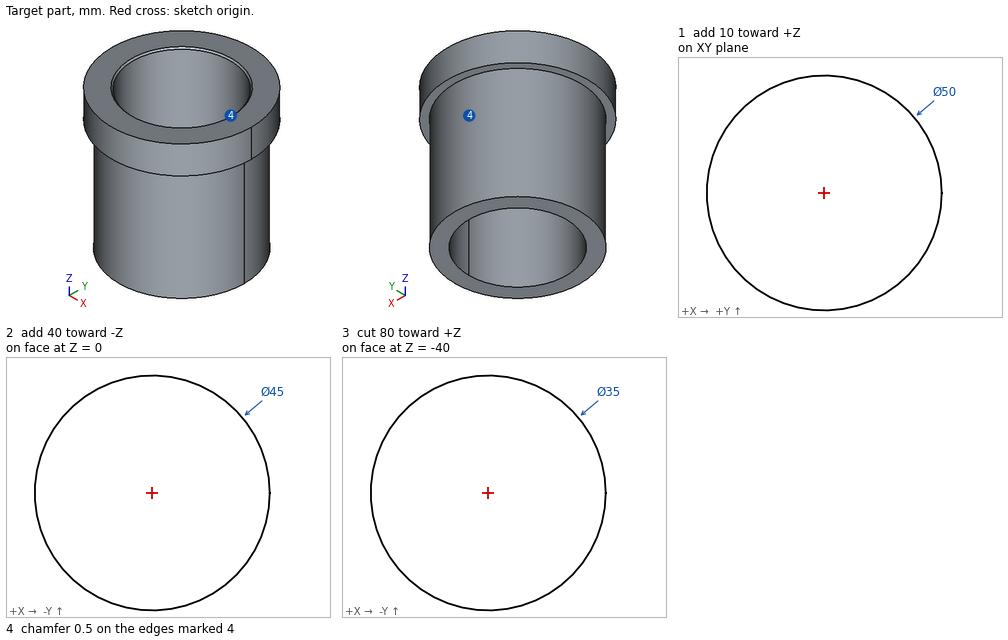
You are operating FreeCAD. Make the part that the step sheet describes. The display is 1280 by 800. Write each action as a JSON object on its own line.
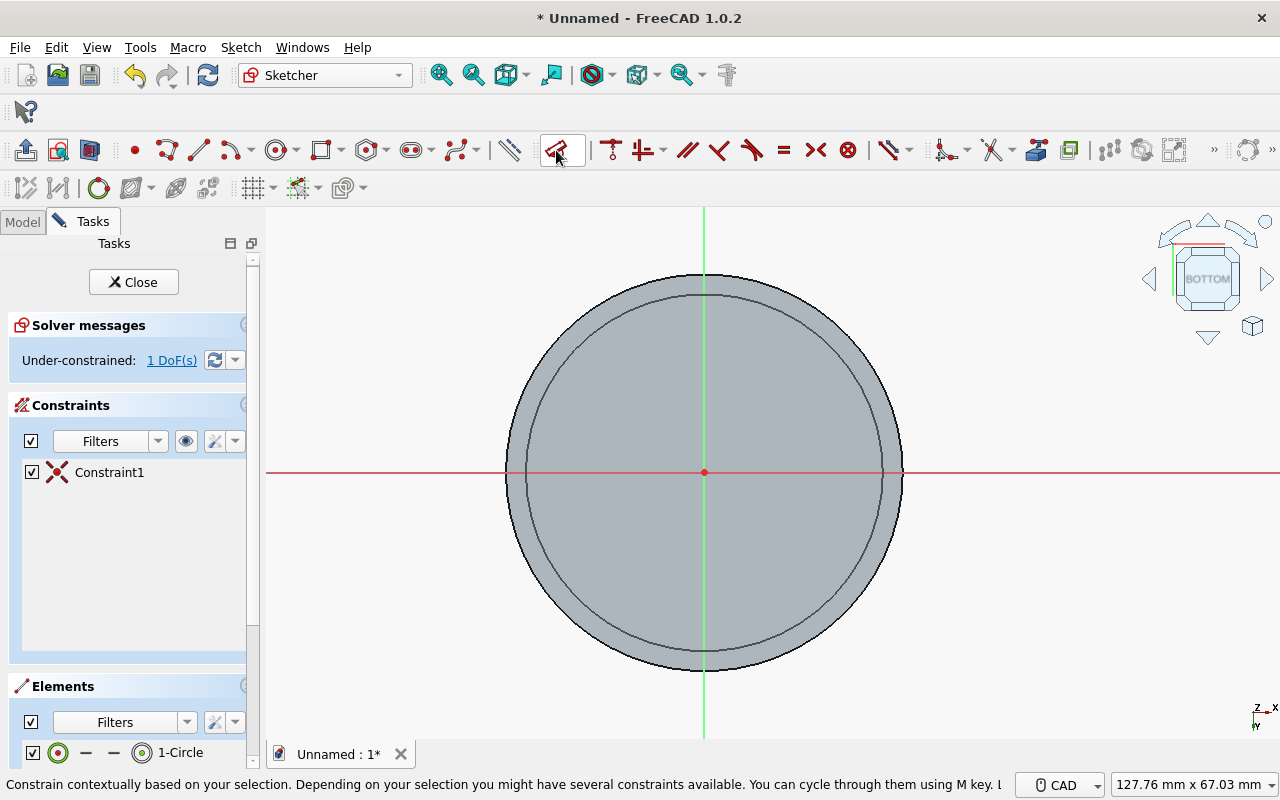
{"action": "left_click", "coordinate": [830, 346]}
{"action": "left_click", "coordinate": [853, 323]}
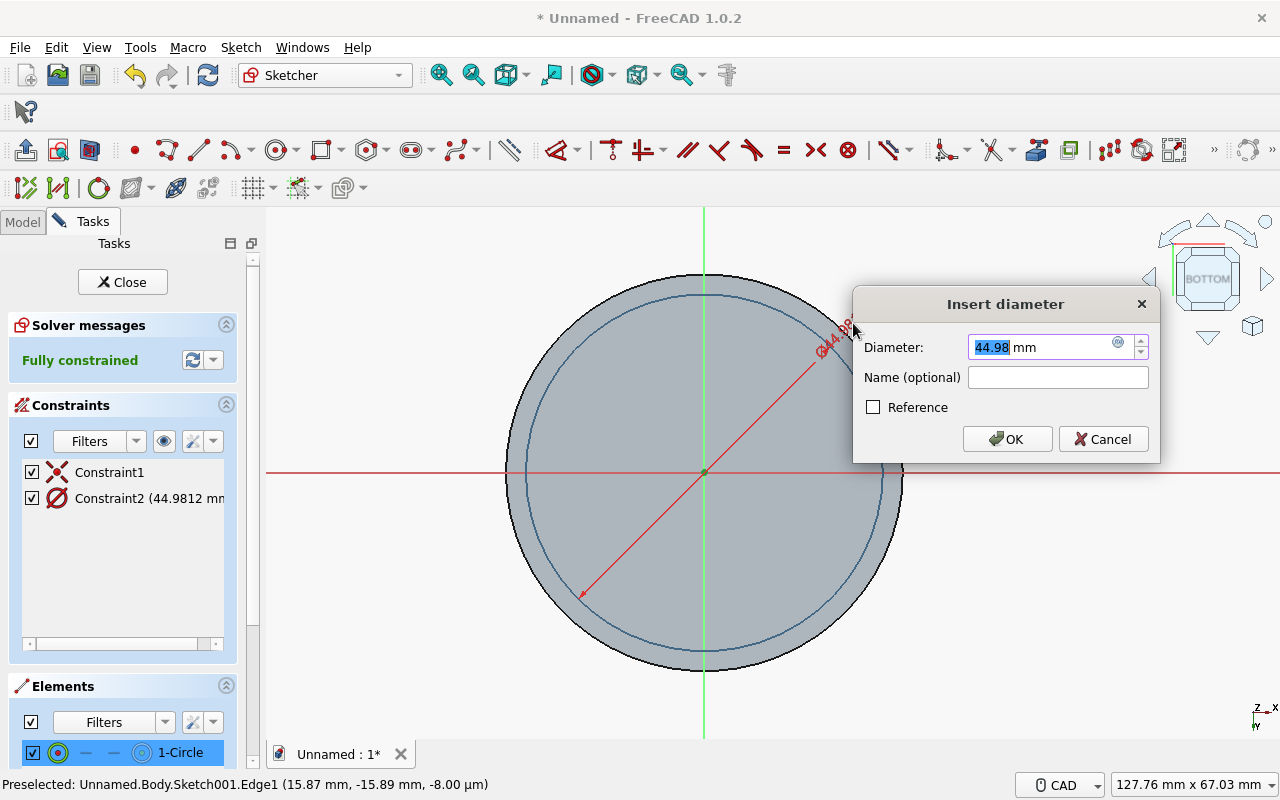
{"action": "type", "text": "45"}
{"action": "key", "text": "Return"}
{"action": "key", "text": "Escape"}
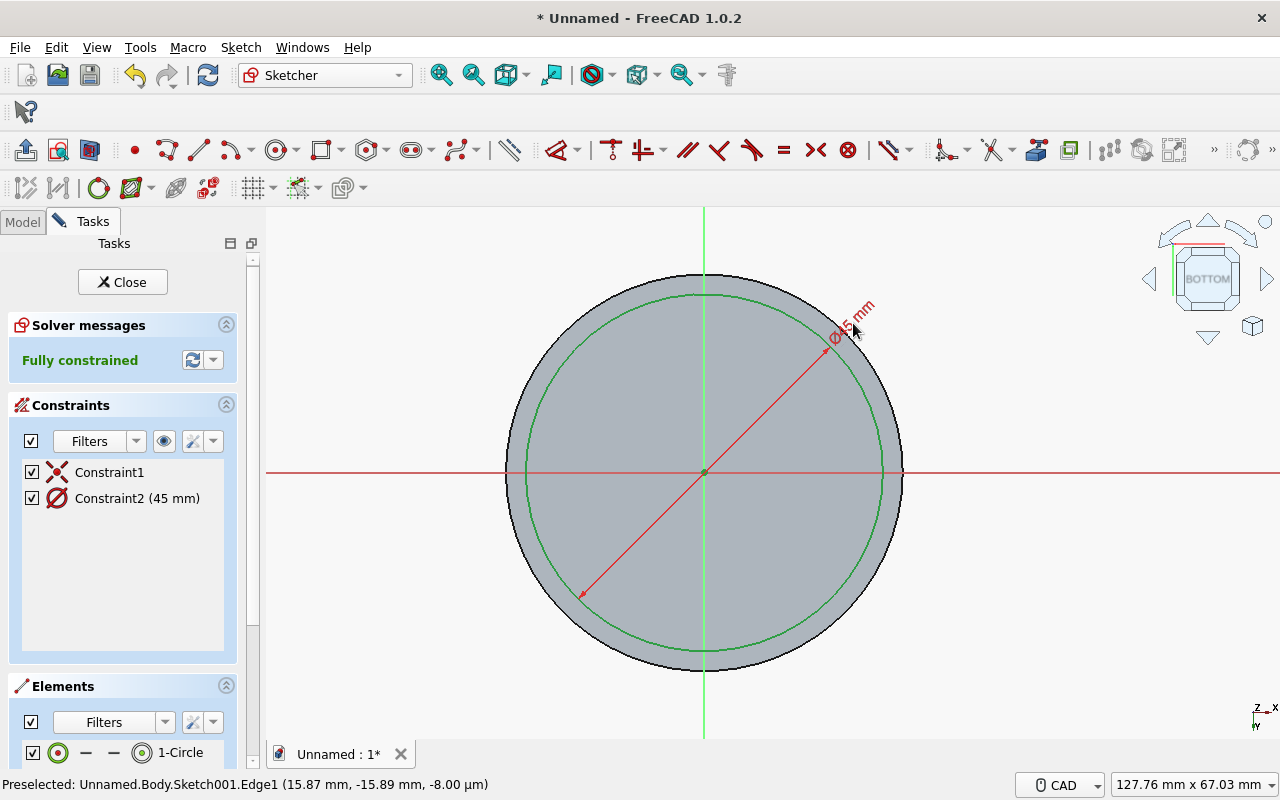
{"action": "left_click", "coordinate": [123, 282]}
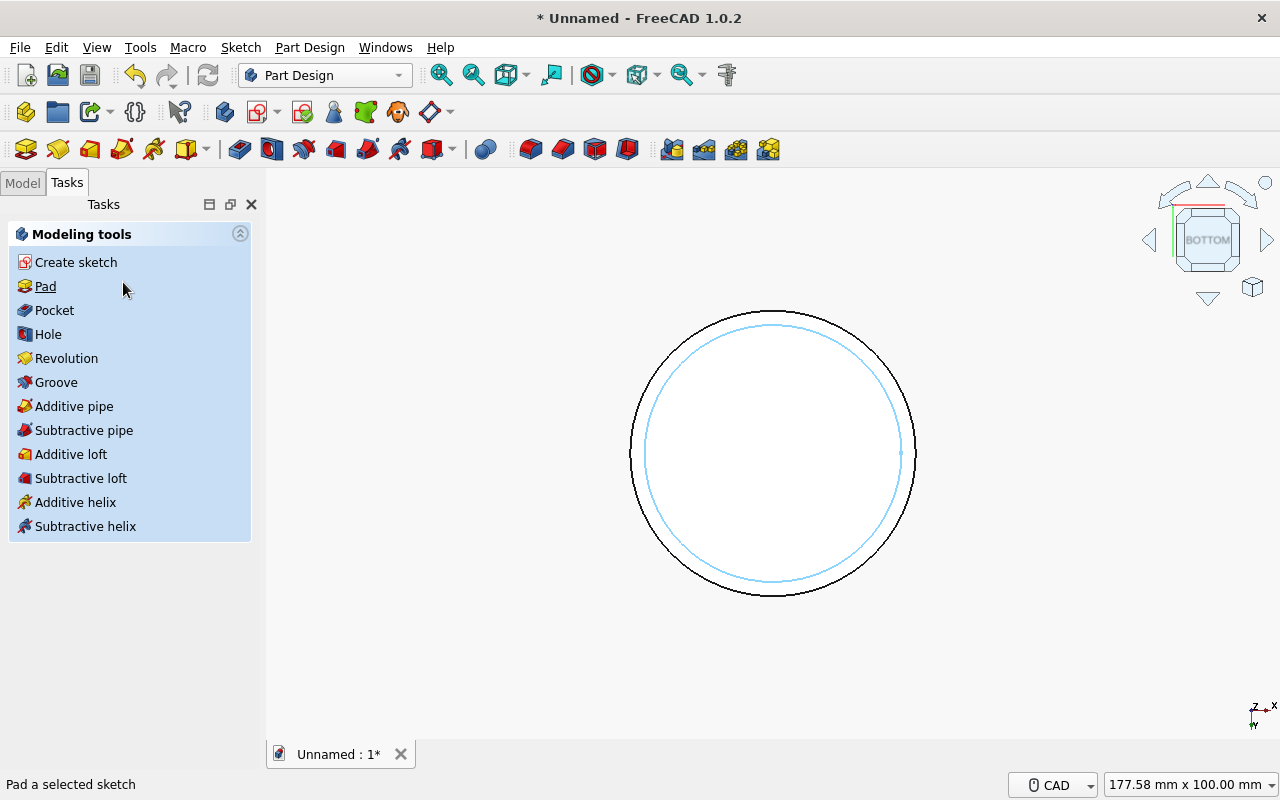
{"action": "left_click", "coordinate": [26, 150]}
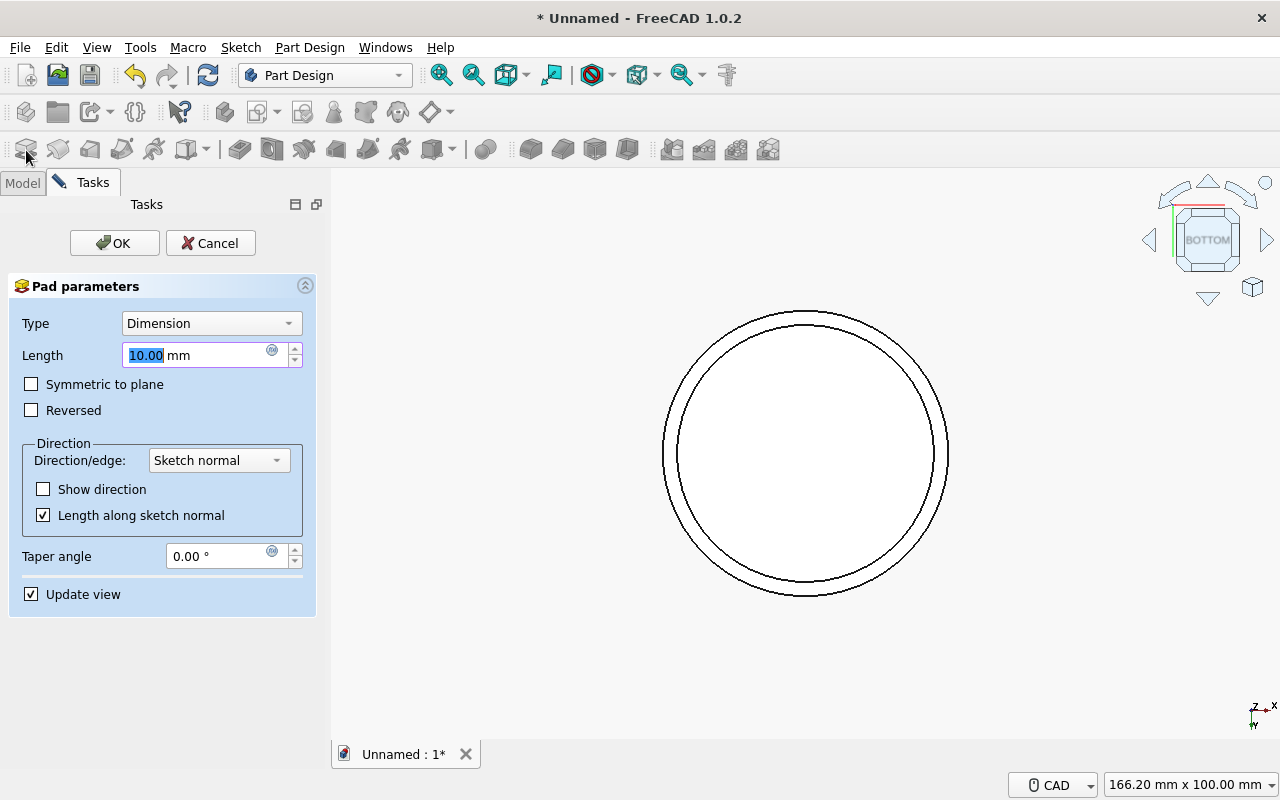
{"action": "type", "text": "40"}
{"action": "key", "text": "Tab"}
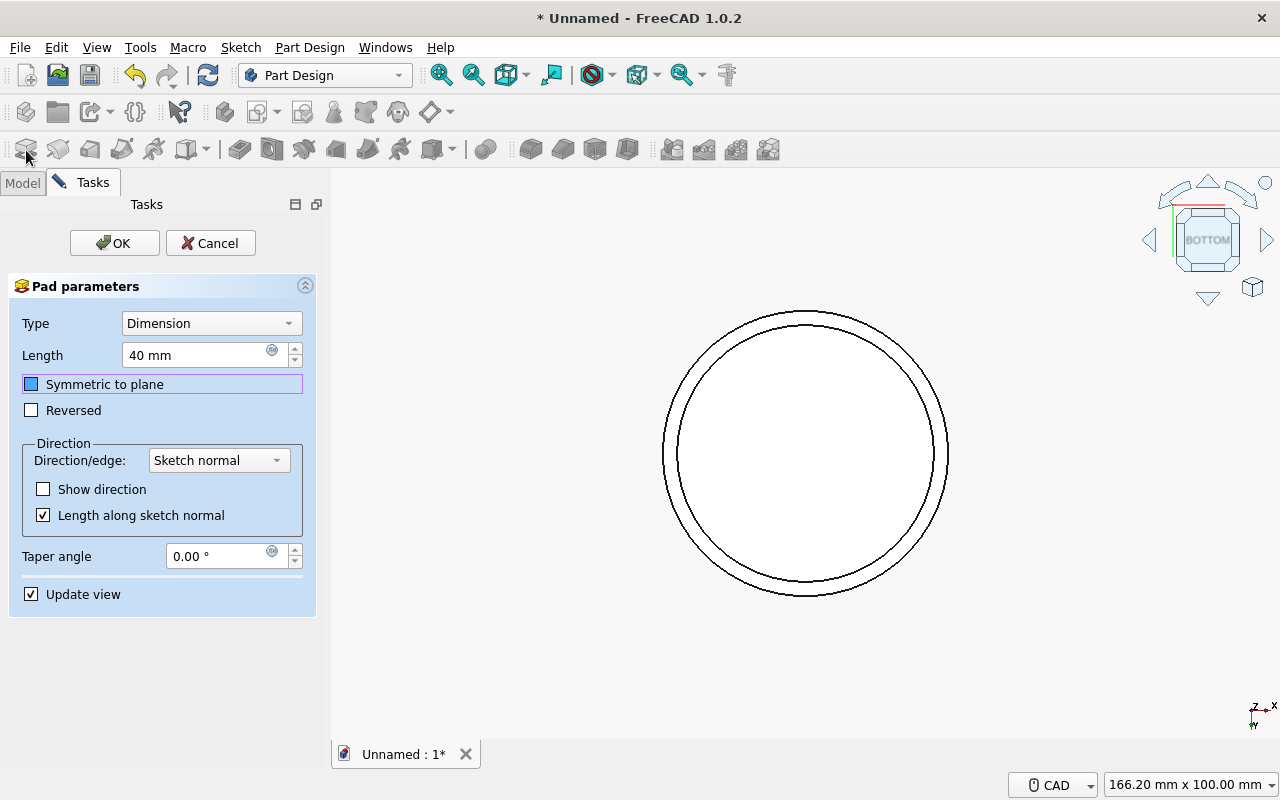
{"action": "left_click", "coordinate": [115, 243]}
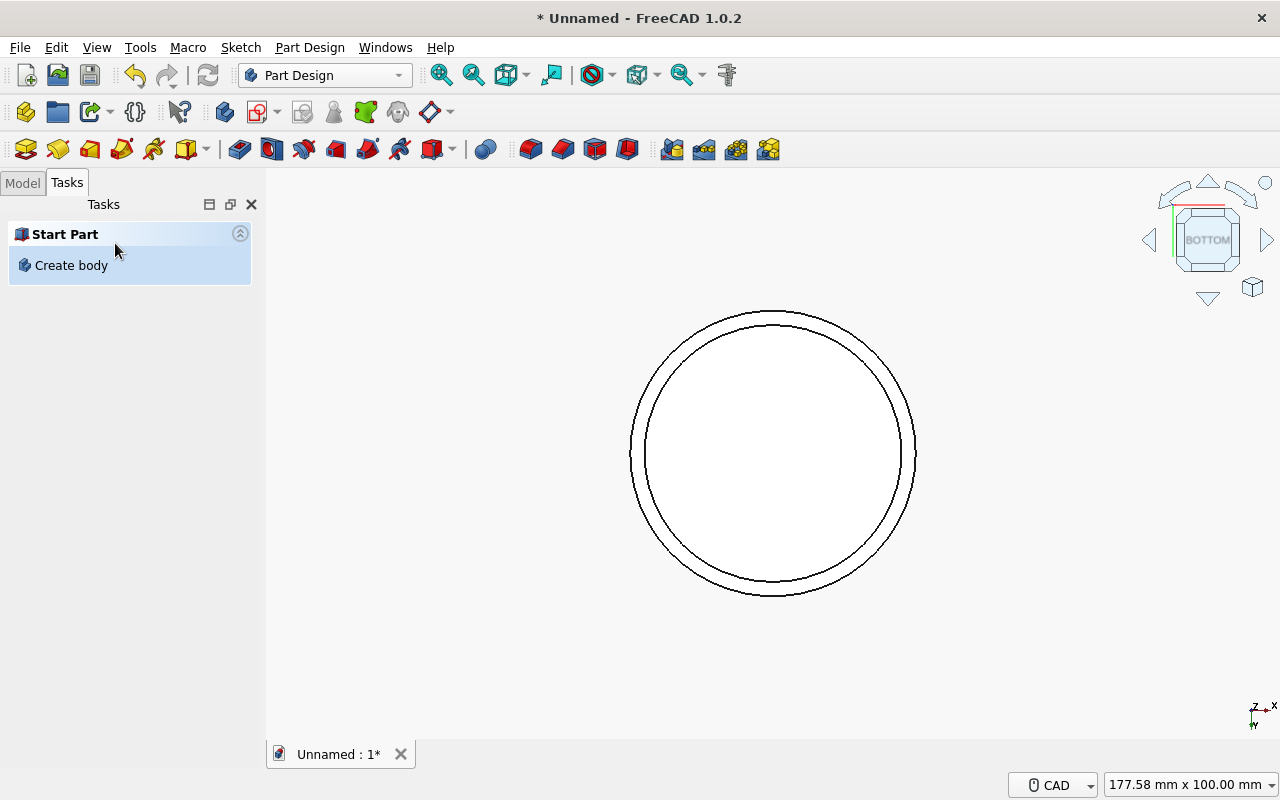
{"action": "left_click", "coordinate": [773, 453]}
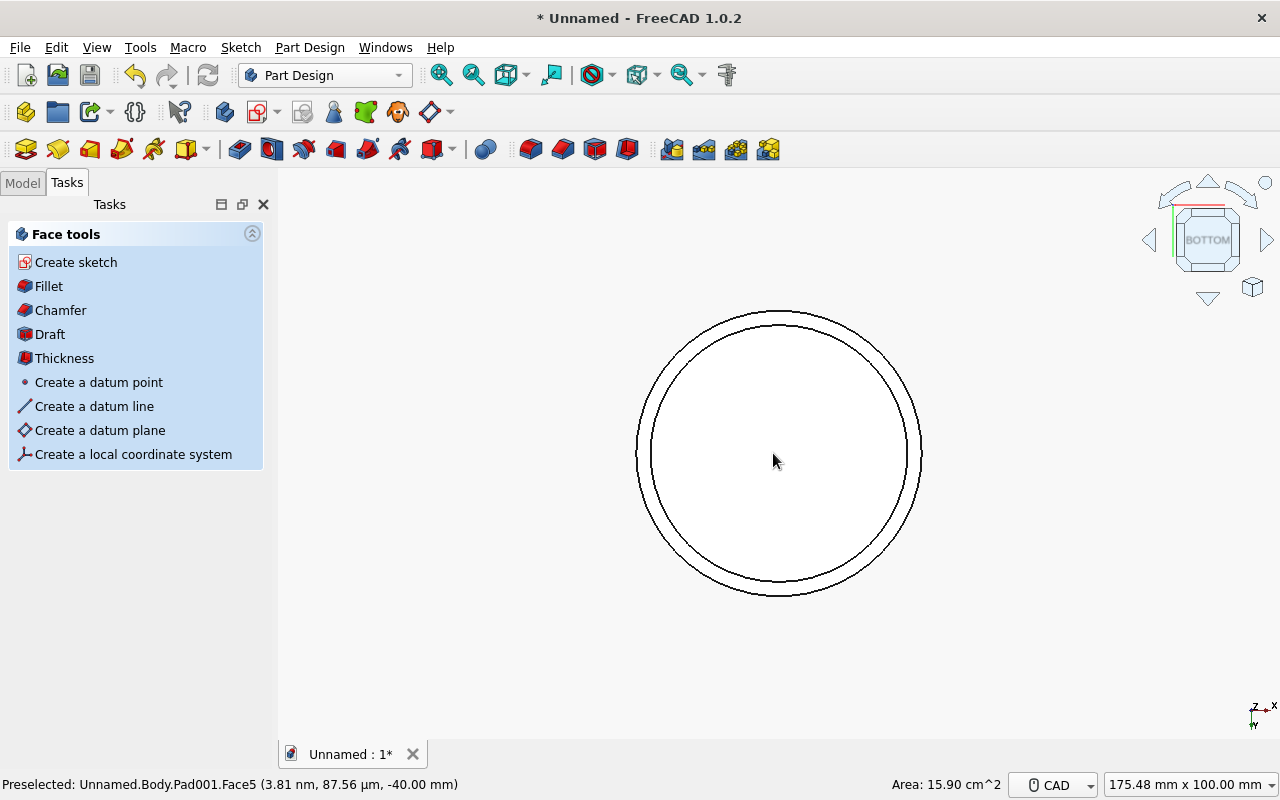
{"action": "left_click", "coordinate": [258, 112]}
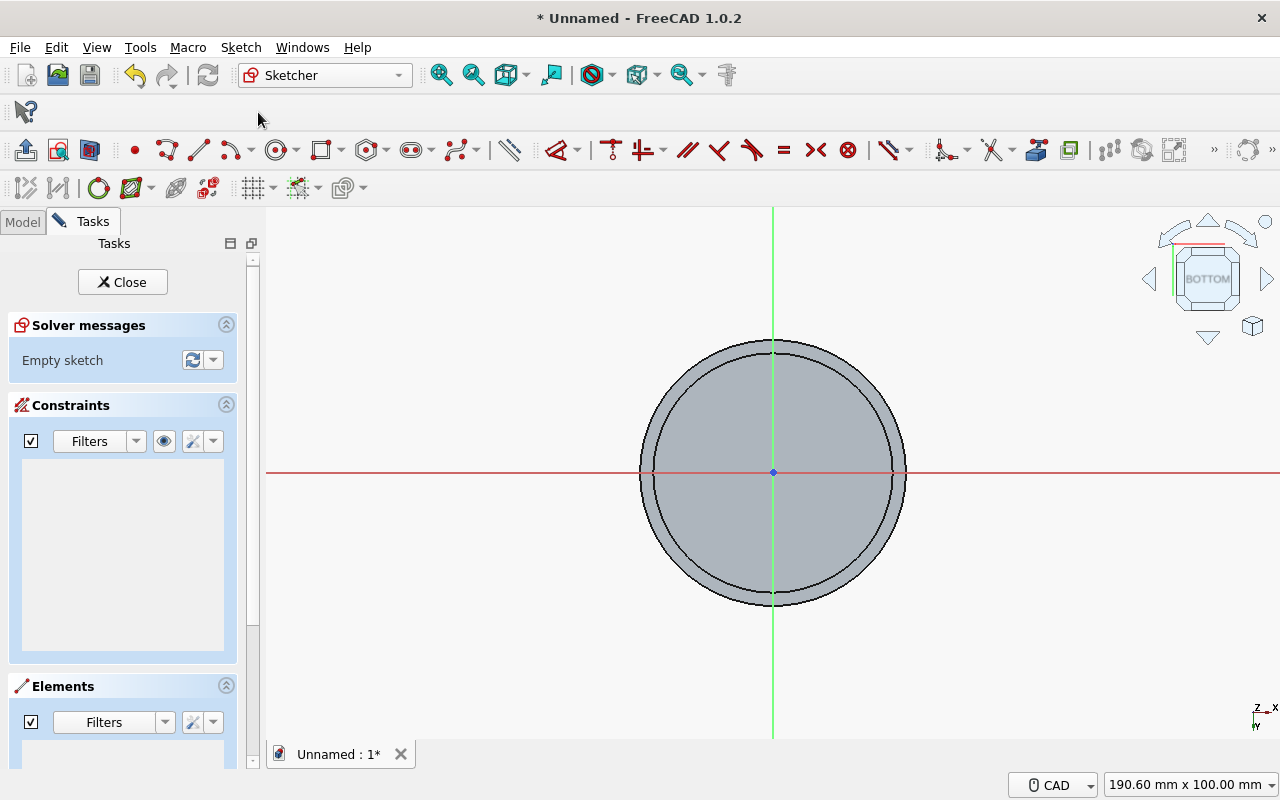
{"action": "scroll", "coordinate": [856, 473], "scroll_direction": "up", "scroll_amount": 3}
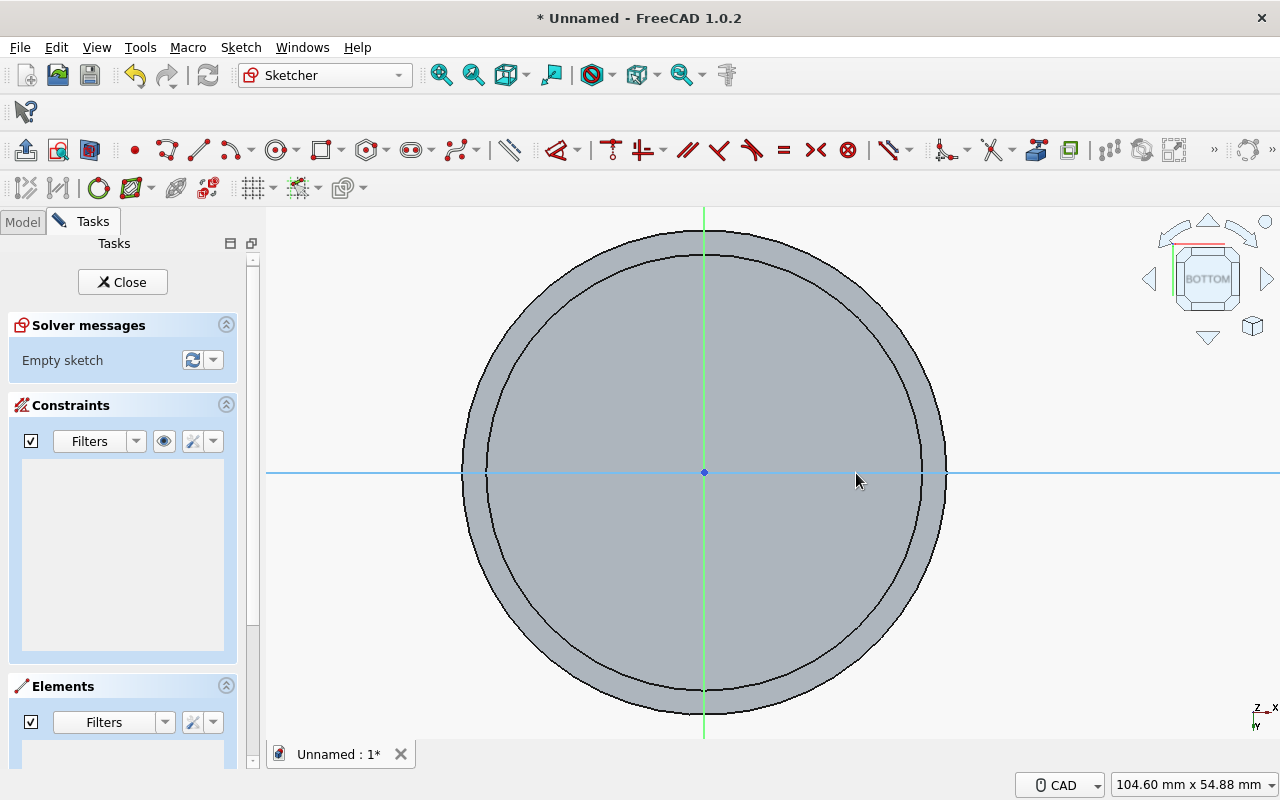
{"action": "key", "text": "g c"}